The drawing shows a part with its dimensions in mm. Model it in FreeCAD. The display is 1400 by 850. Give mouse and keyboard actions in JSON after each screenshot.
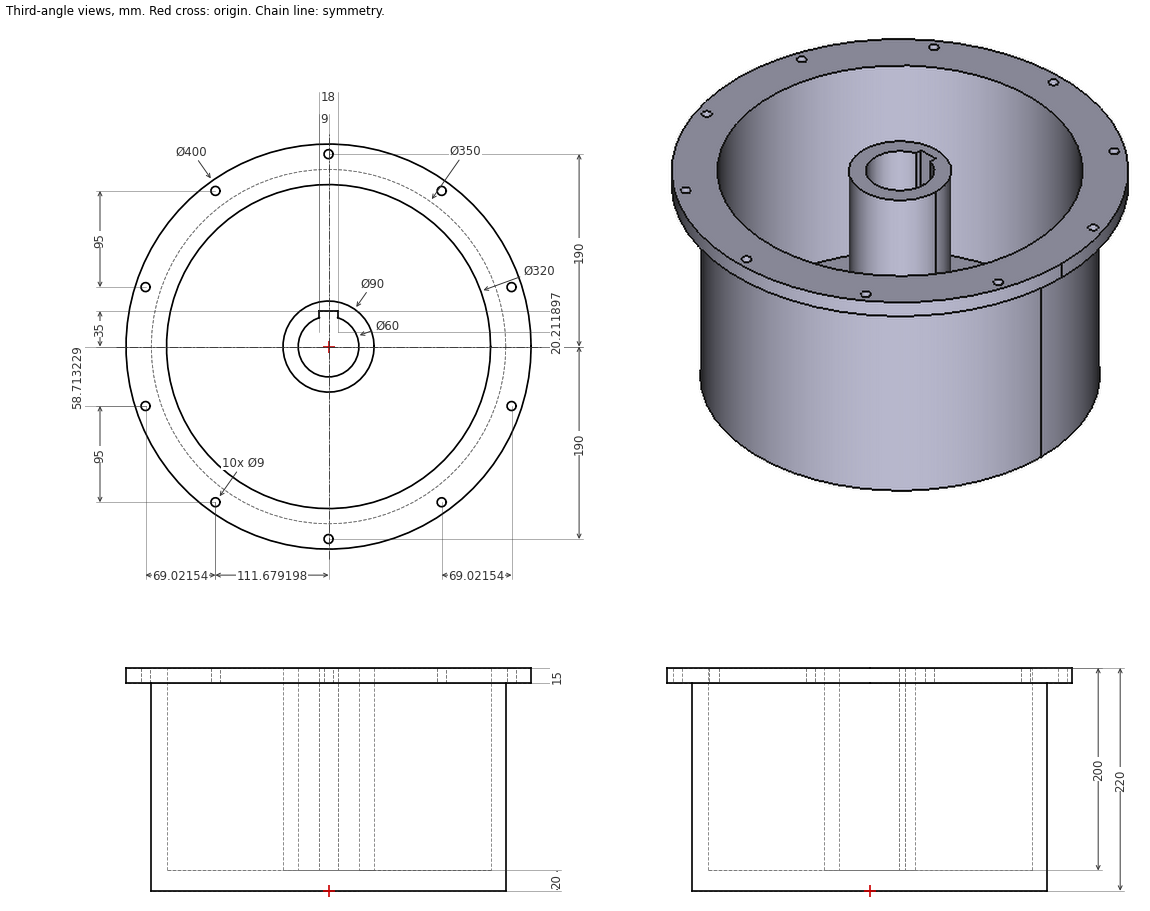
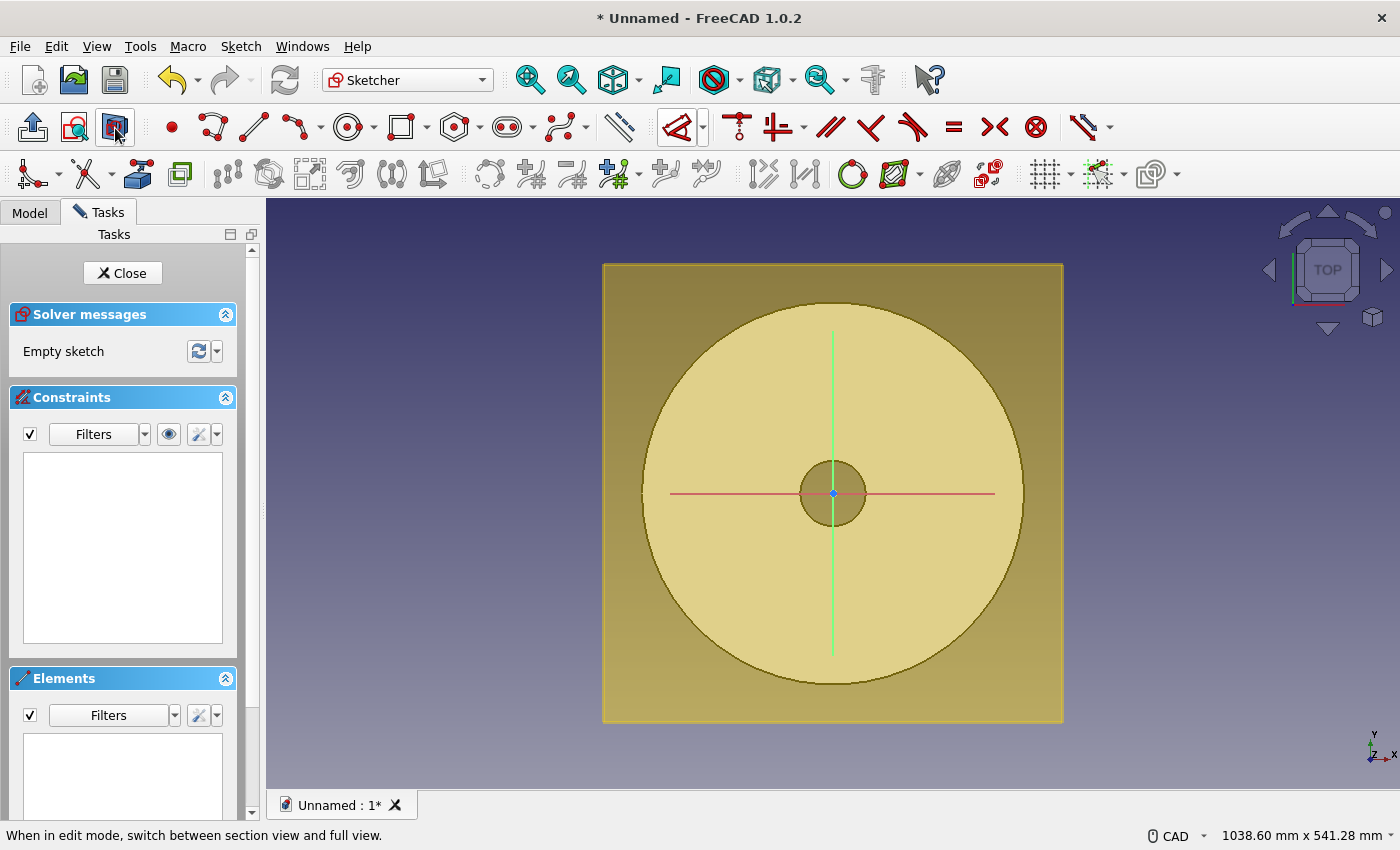
{"action": "left_click", "coordinate": [348, 128]}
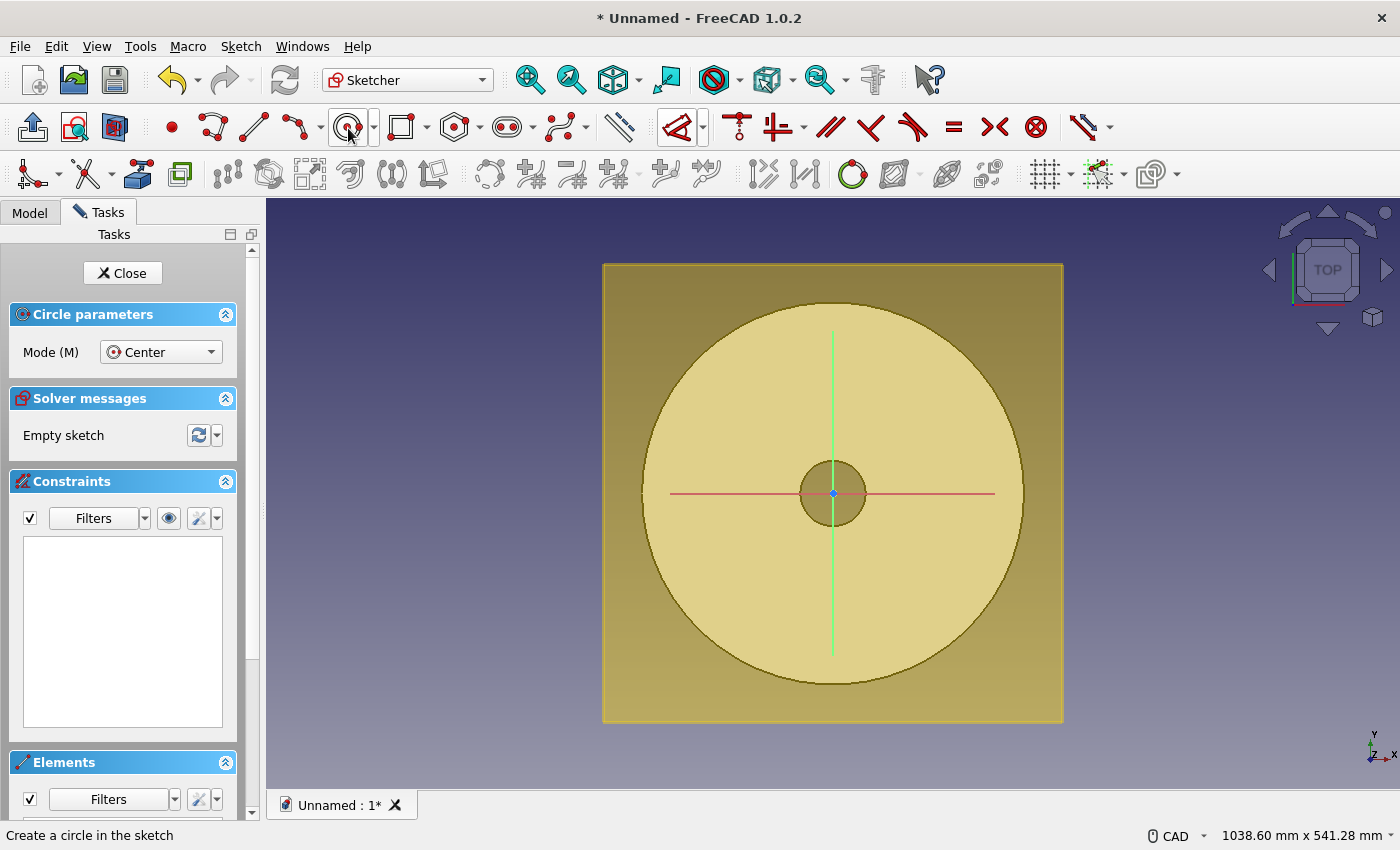
{"action": "left_click", "coordinate": [833, 494]}
{"action": "mouse_move", "coordinate": [987, 339]}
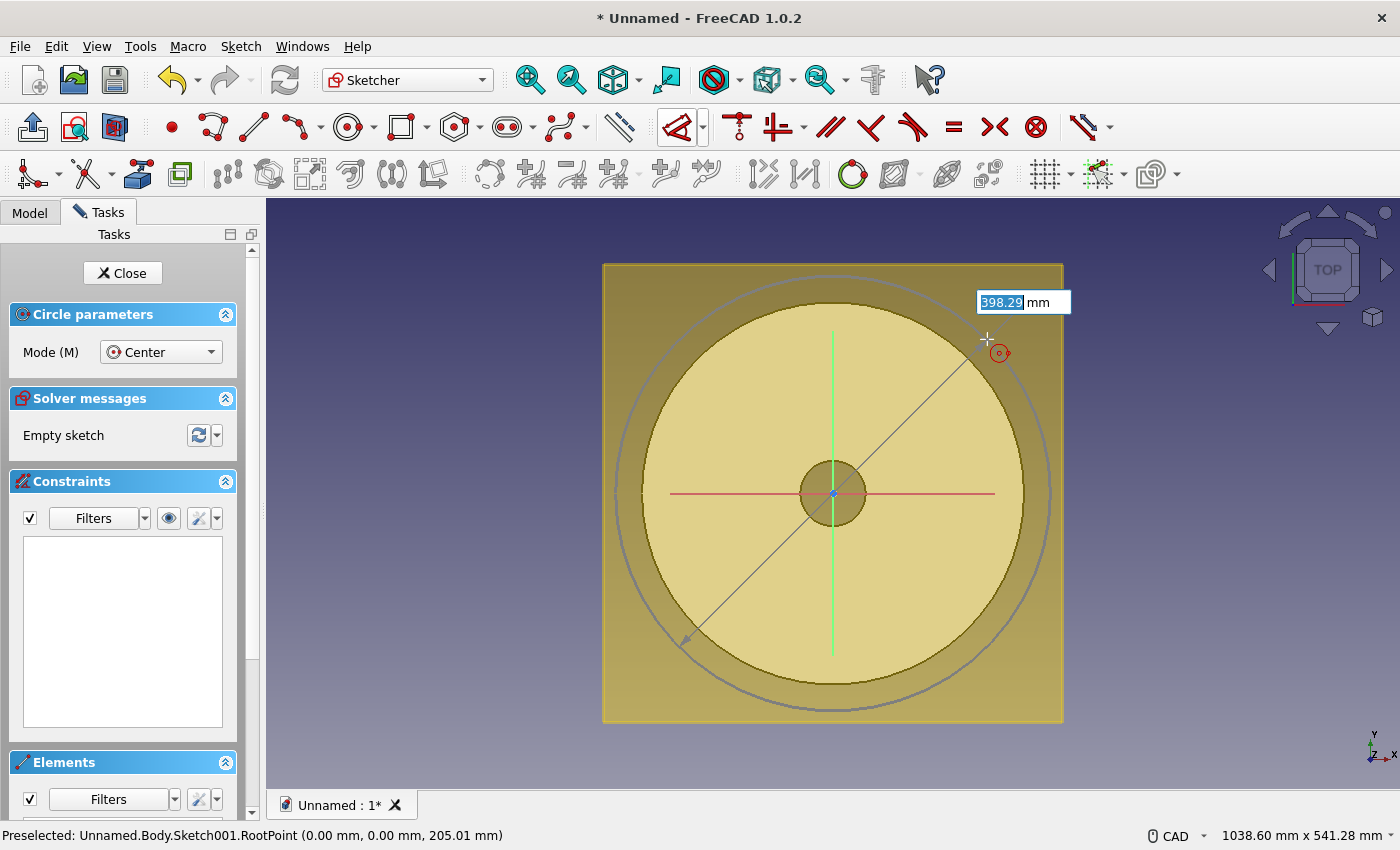
{"action": "type", "text": "400"}
{"action": "key", "text": "Return"}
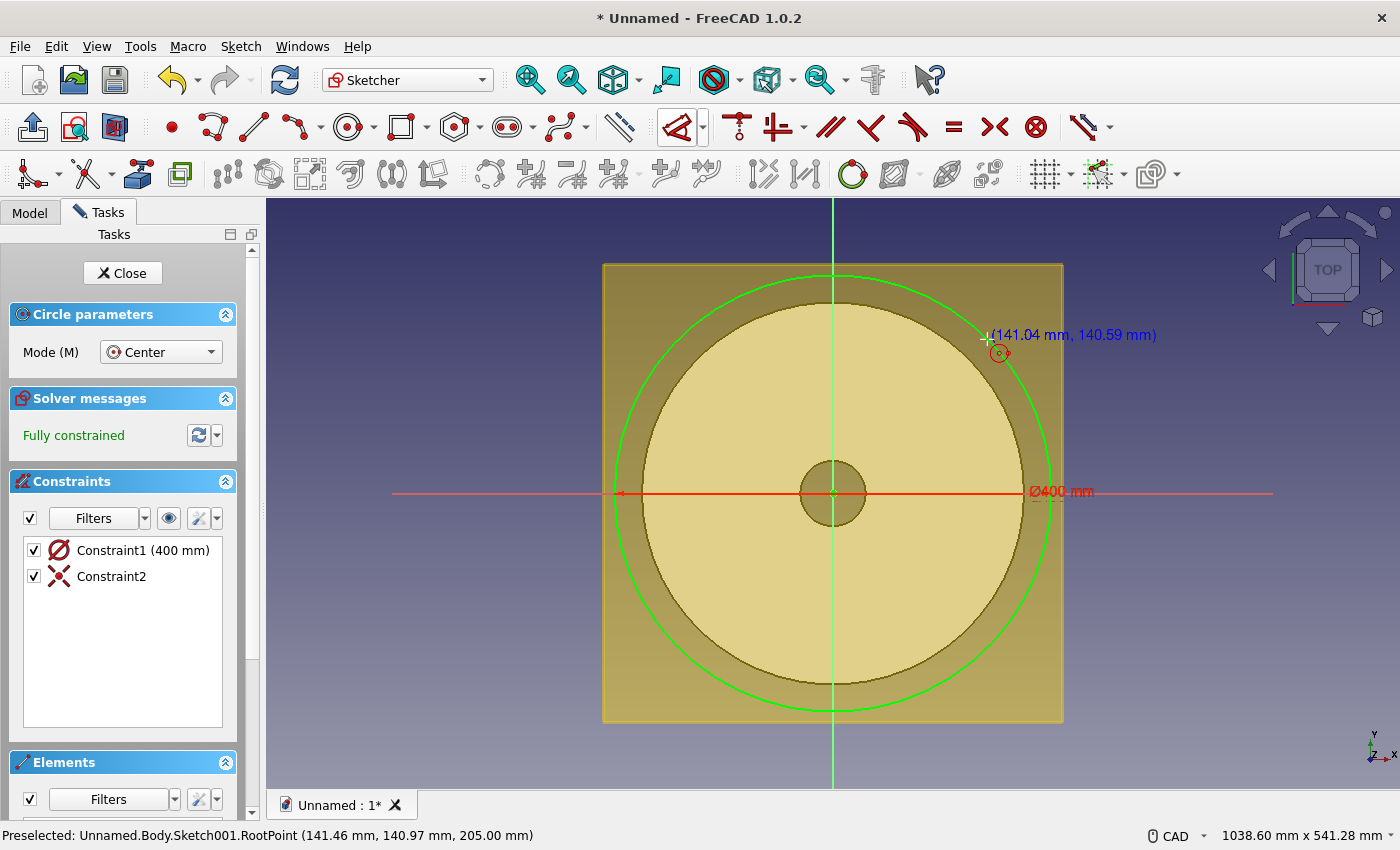
{"action": "scroll", "coordinate": [711, 661], "scroll_direction": "up", "scroll_amount": 8}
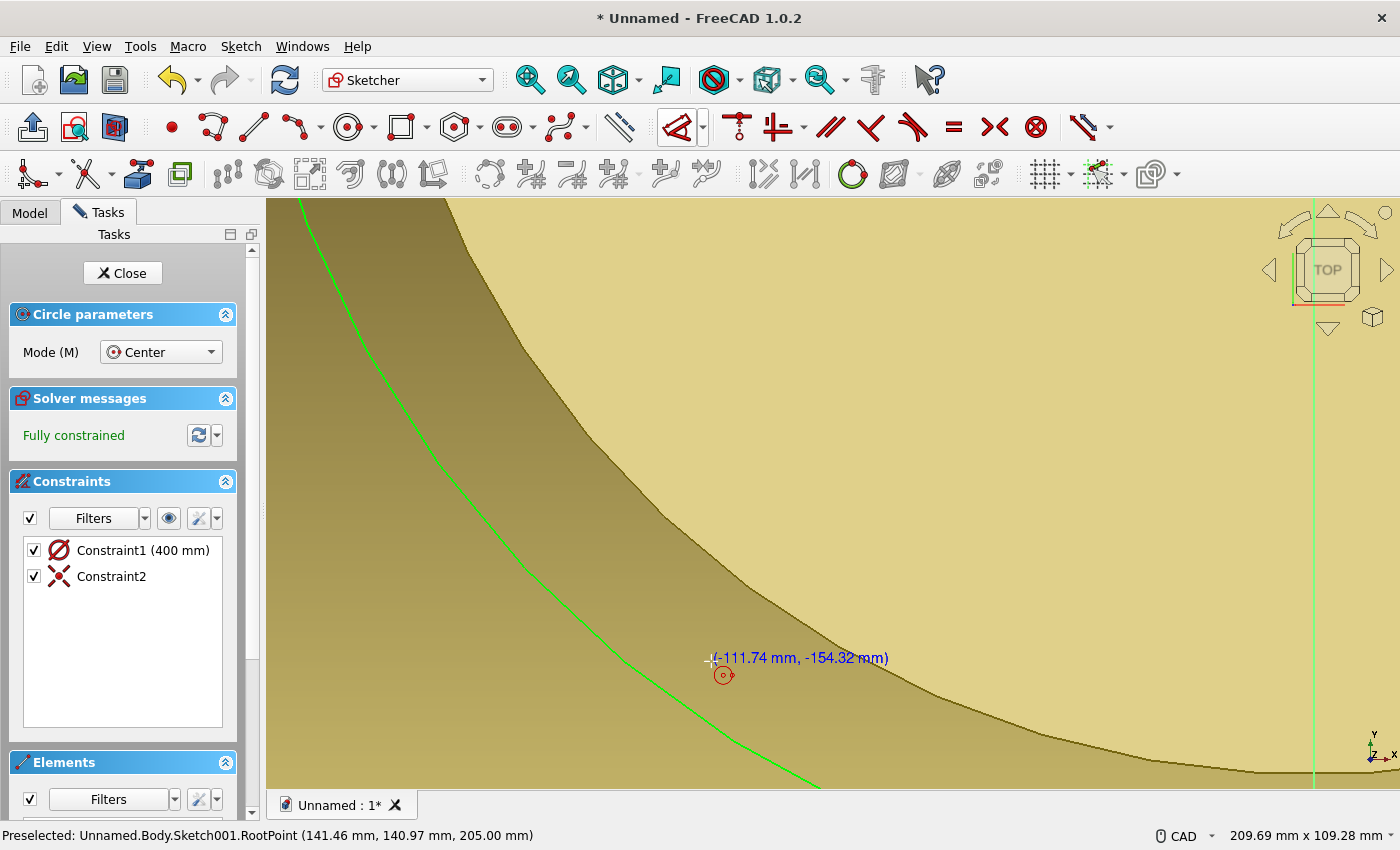
{"action": "scroll", "coordinate": [656, 625], "scroll_direction": "down", "scroll_amount": 9}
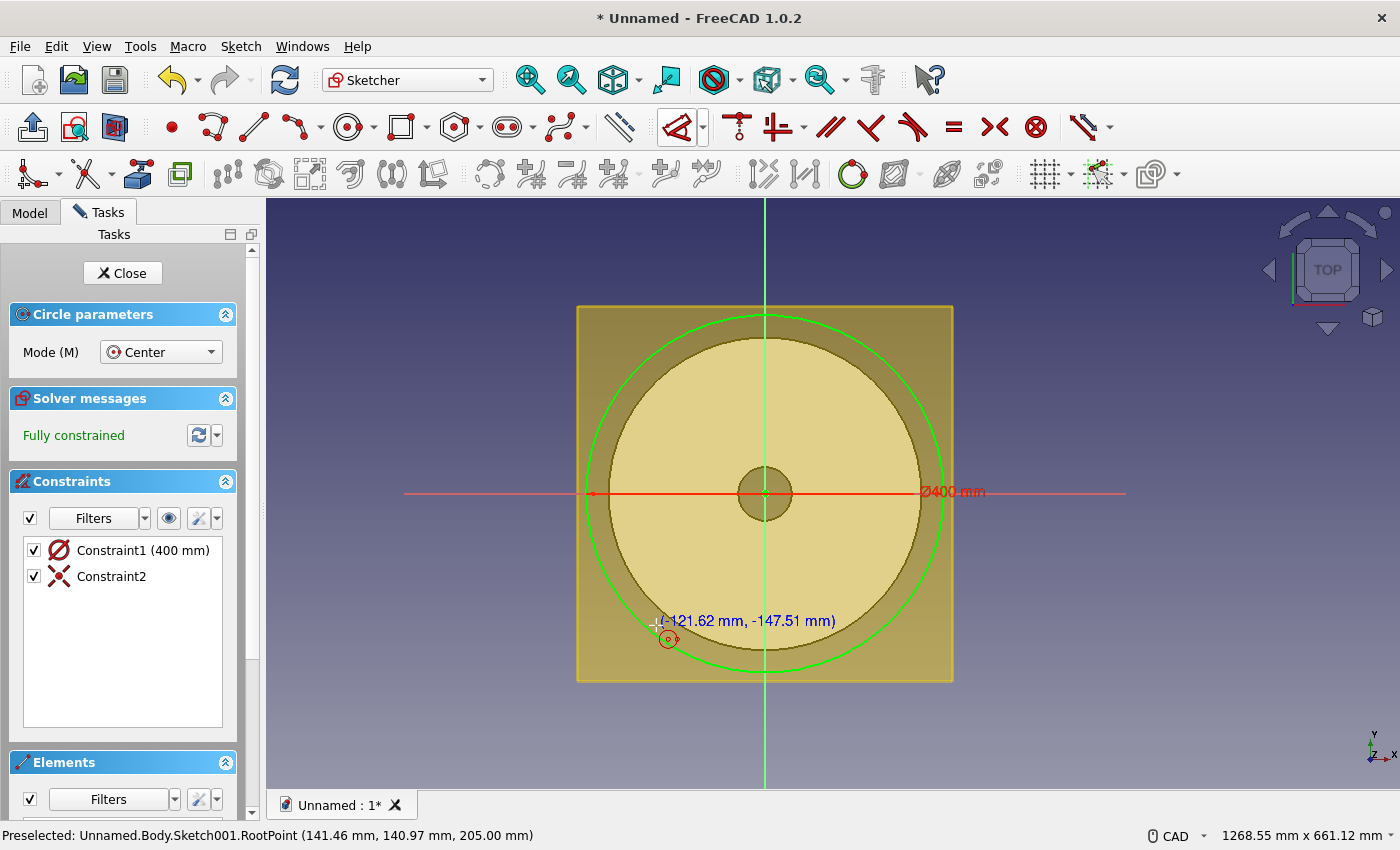
{"action": "scroll", "coordinate": [665, 631], "scroll_direction": "up", "scroll_amount": 3}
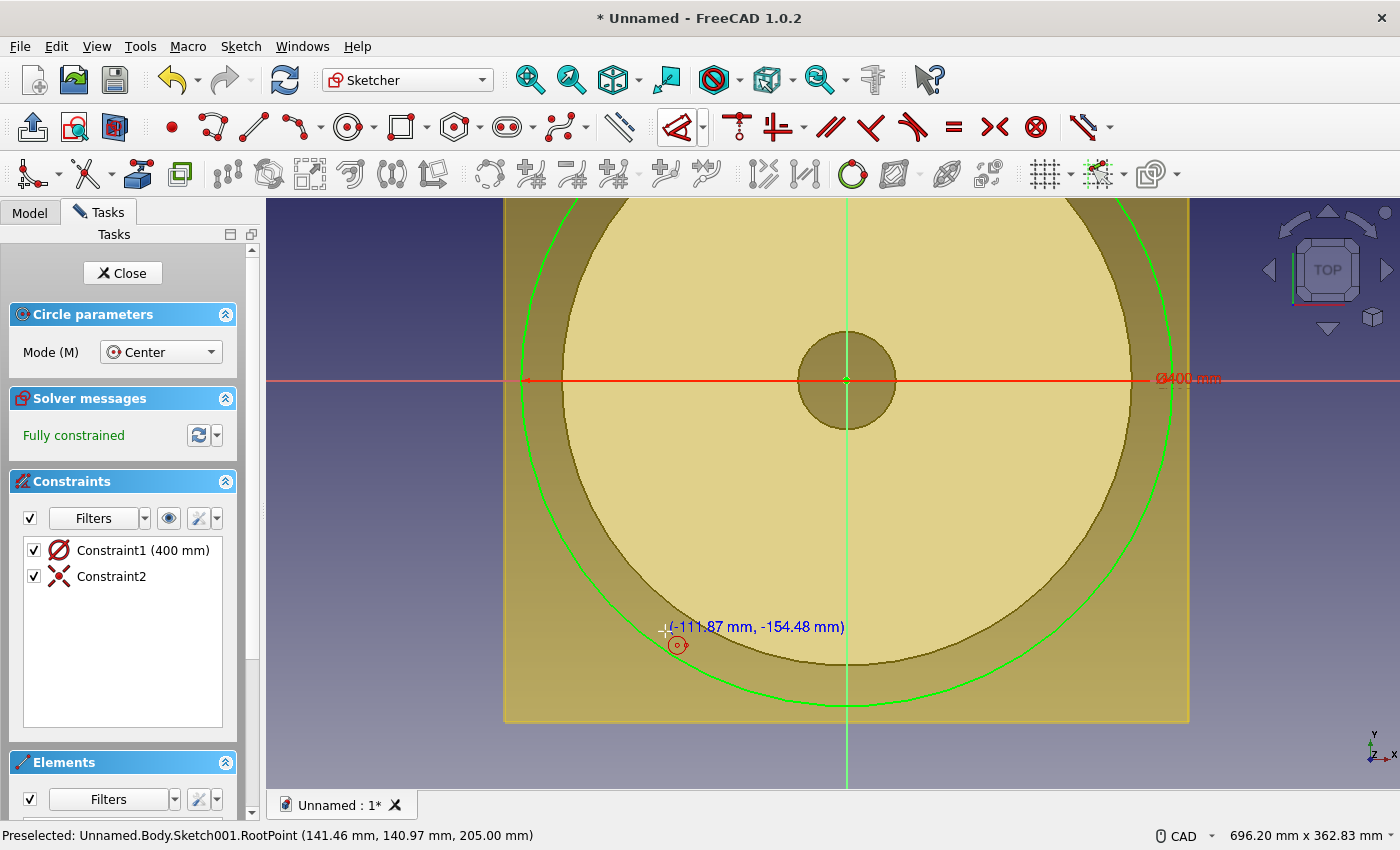
{"action": "left_click", "coordinate": [665, 631]}
{"action": "mouse_move", "coordinate": [670, 626]}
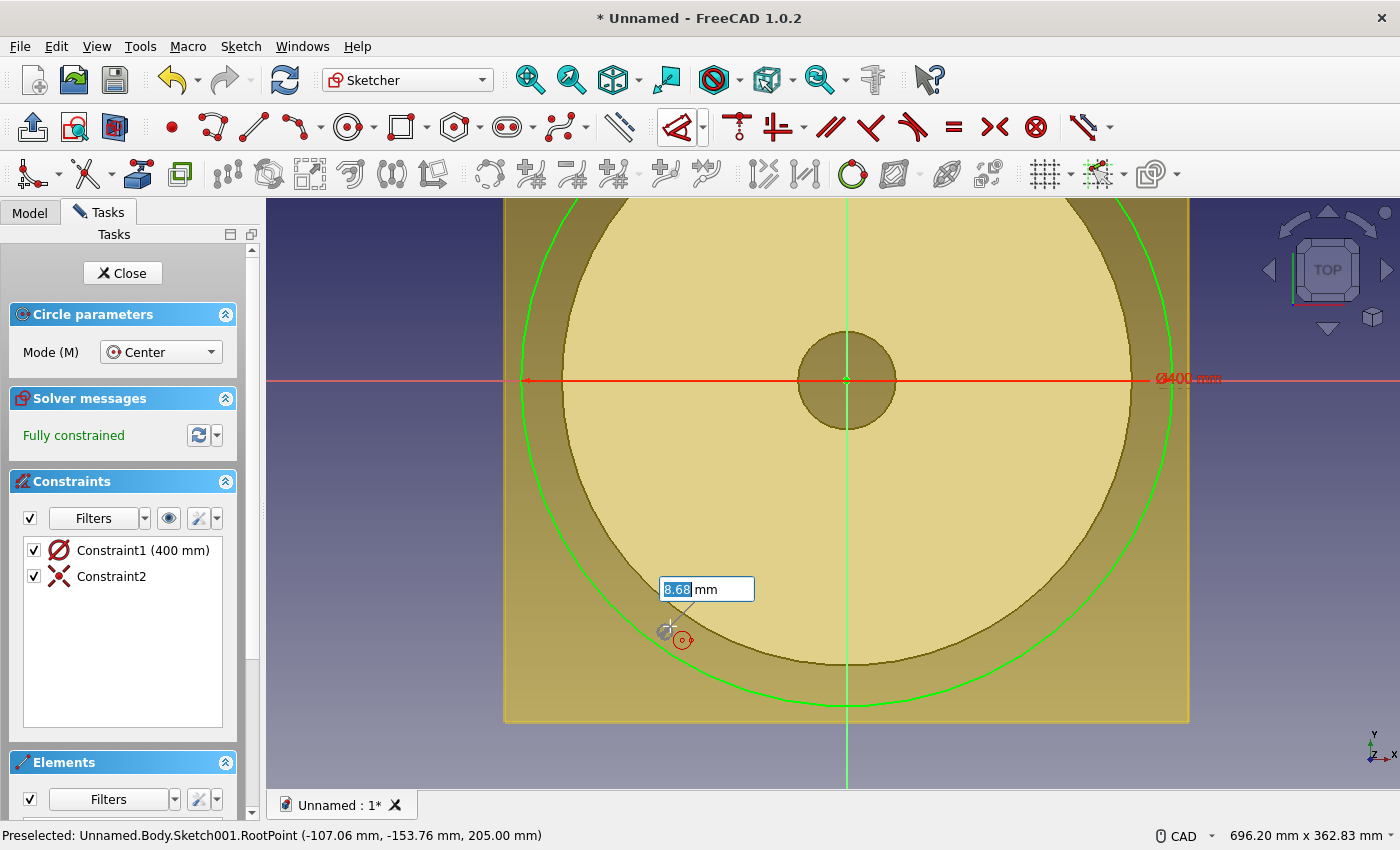
{"action": "type", "text": "9"}
{"action": "key", "text": "Return"}